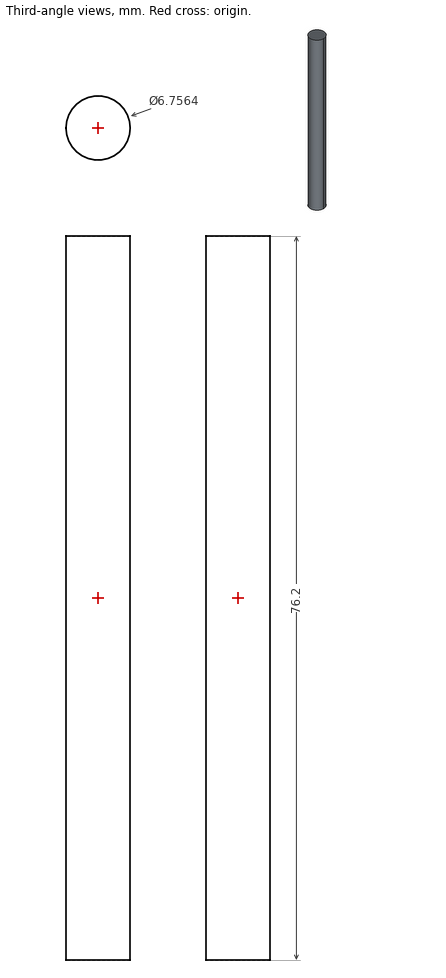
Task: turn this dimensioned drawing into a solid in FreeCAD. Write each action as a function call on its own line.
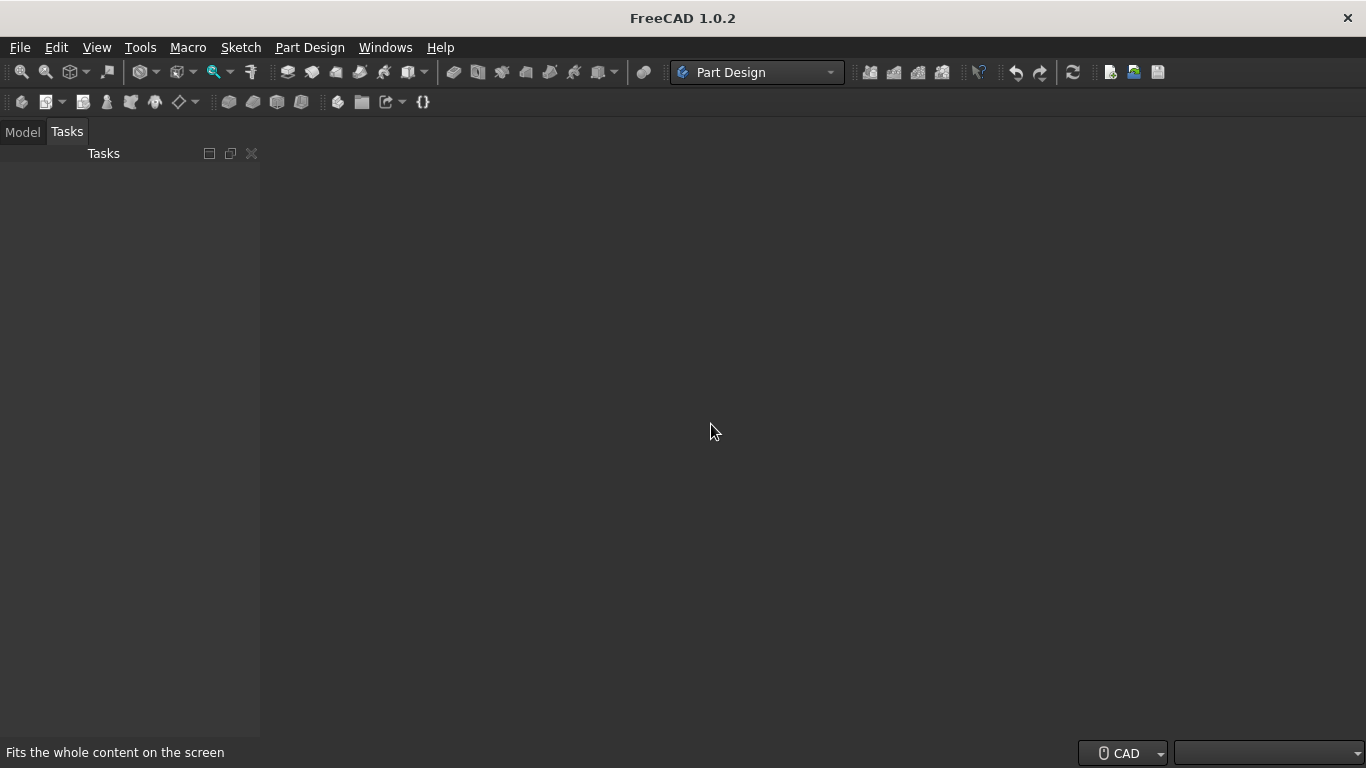
click(1110, 72)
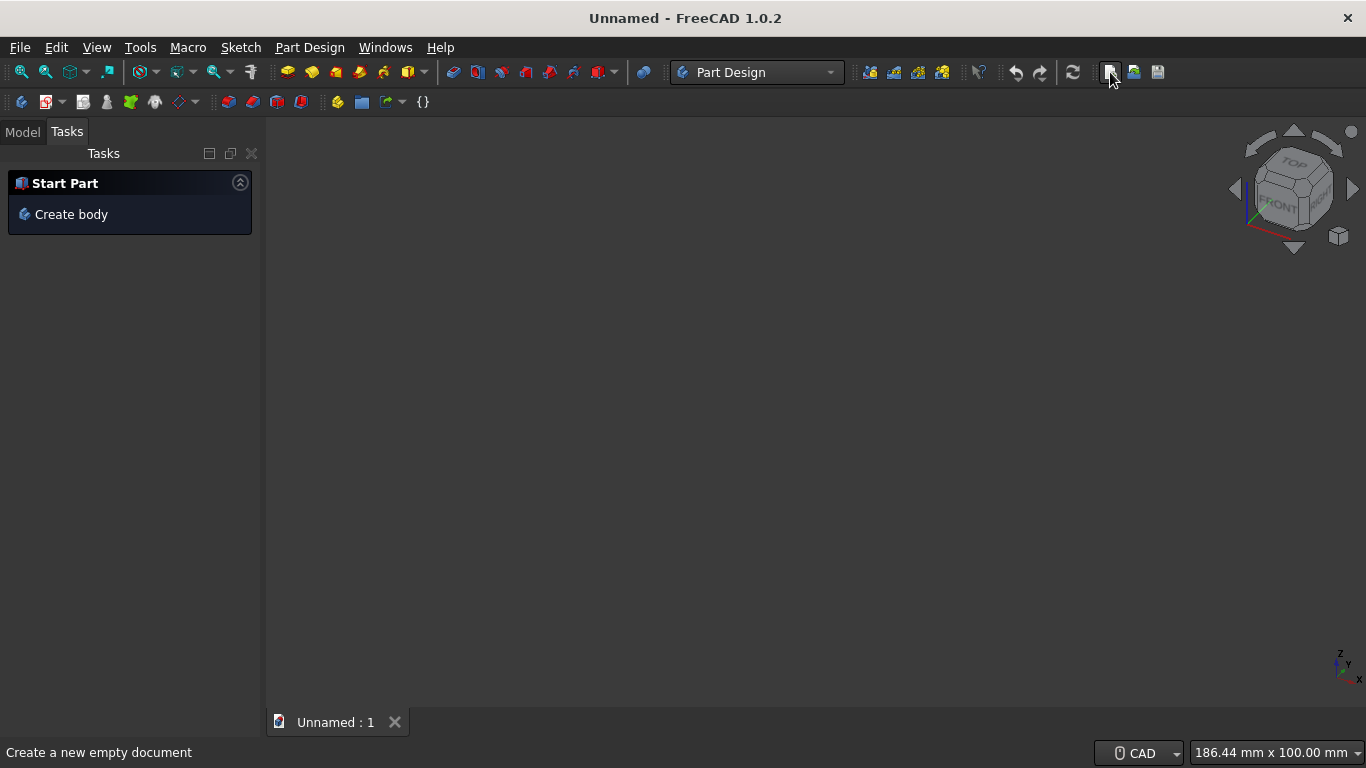
click(46, 102)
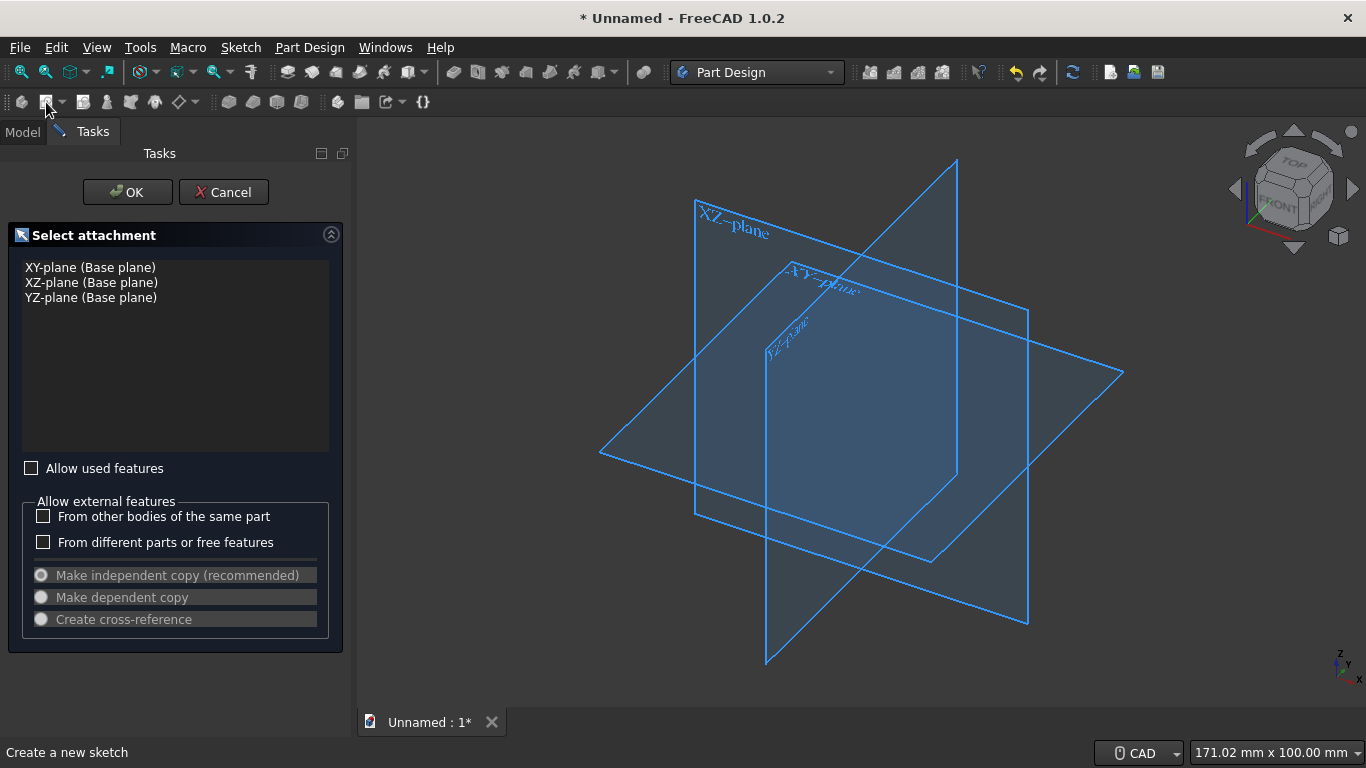
click(82, 268)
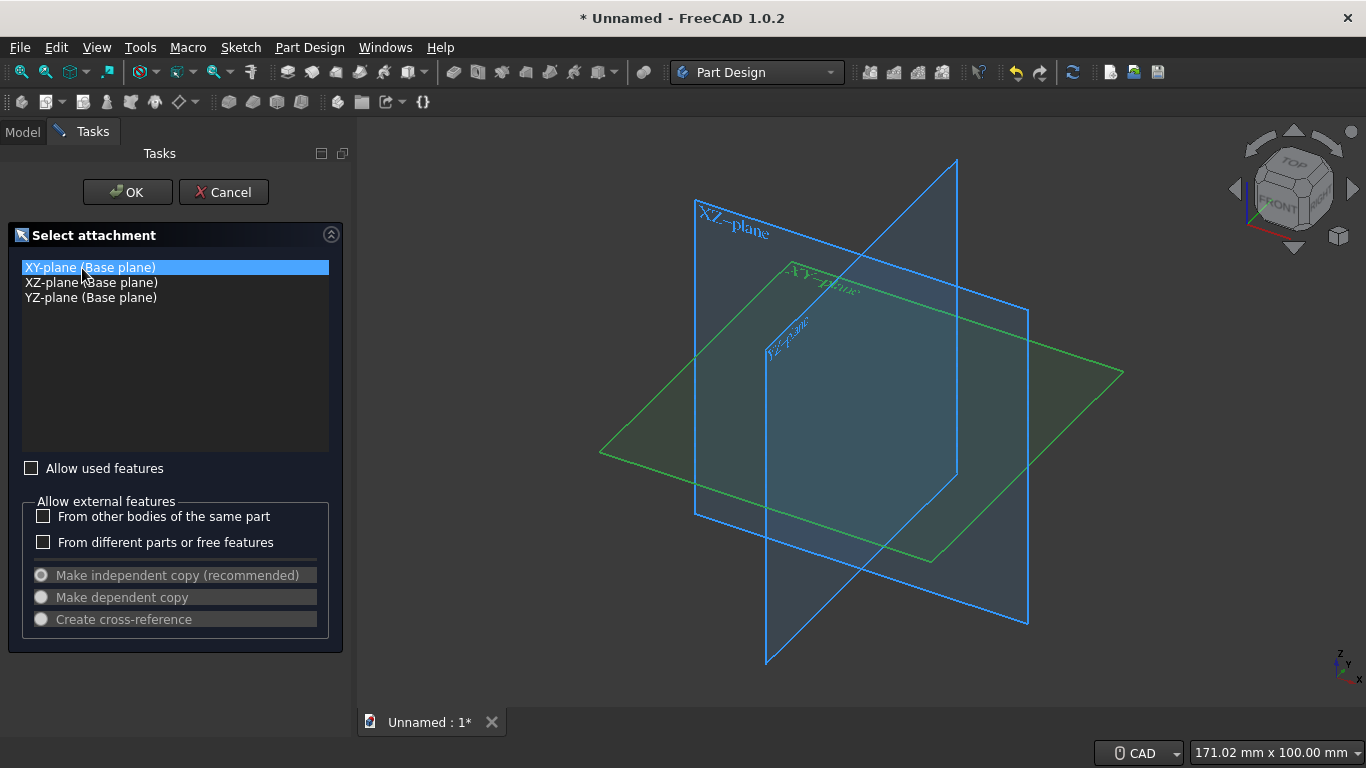
click(128, 192)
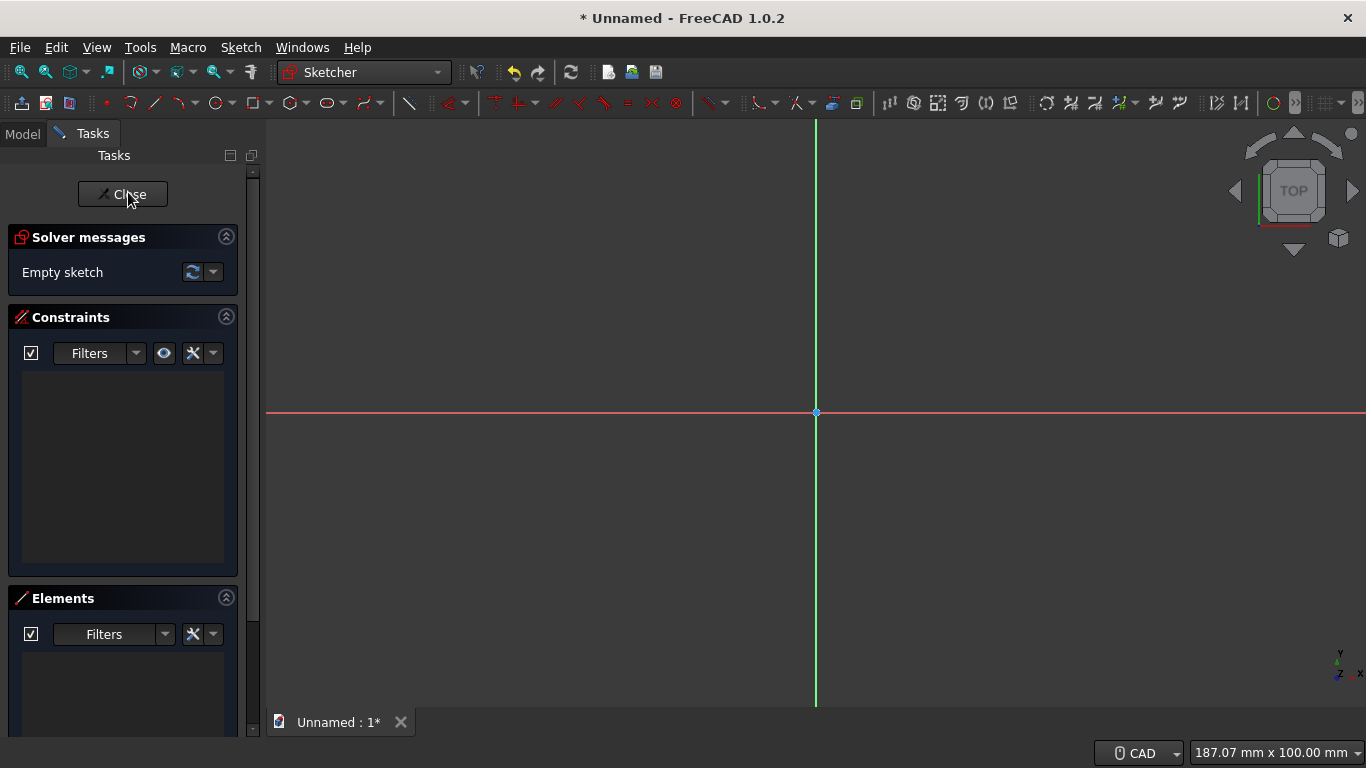
scroll(825, 413, up, 11)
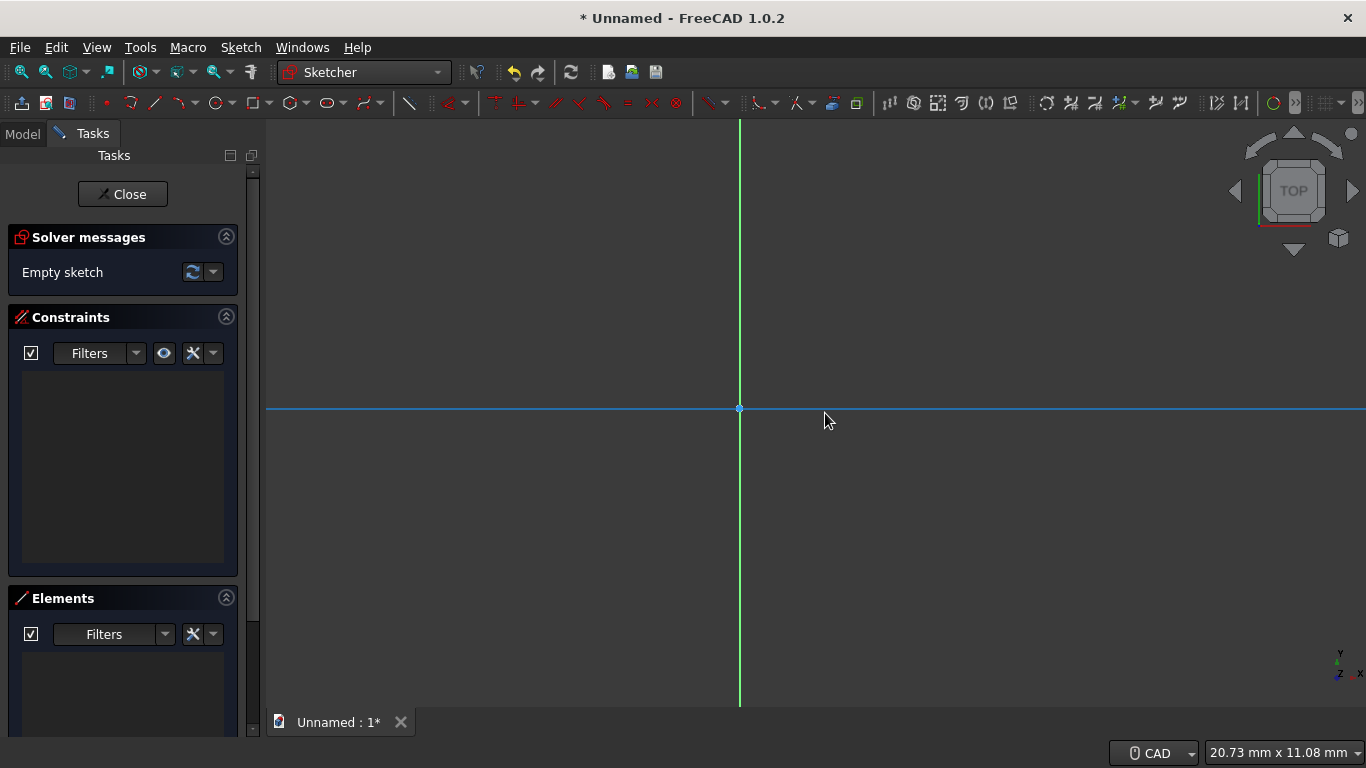
click(216, 104)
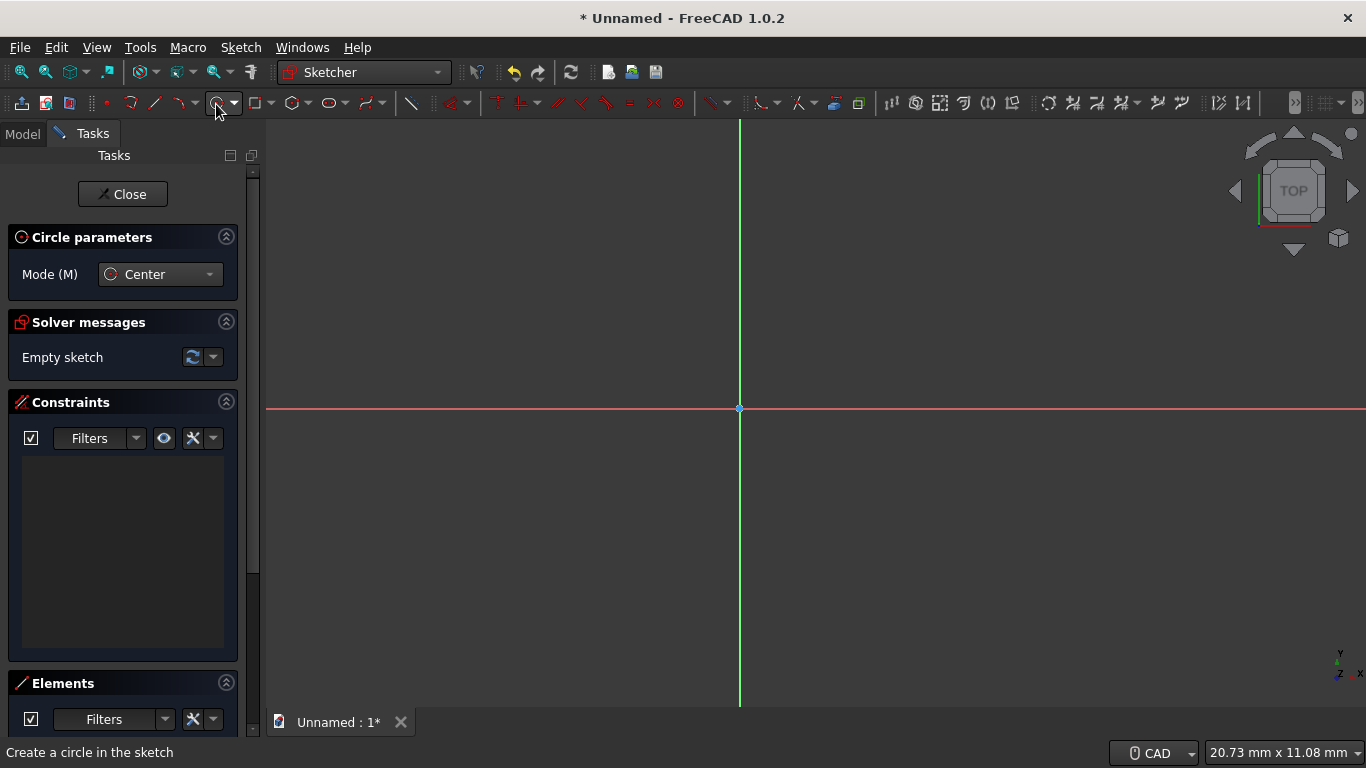
click(740, 409)
move(866, 282)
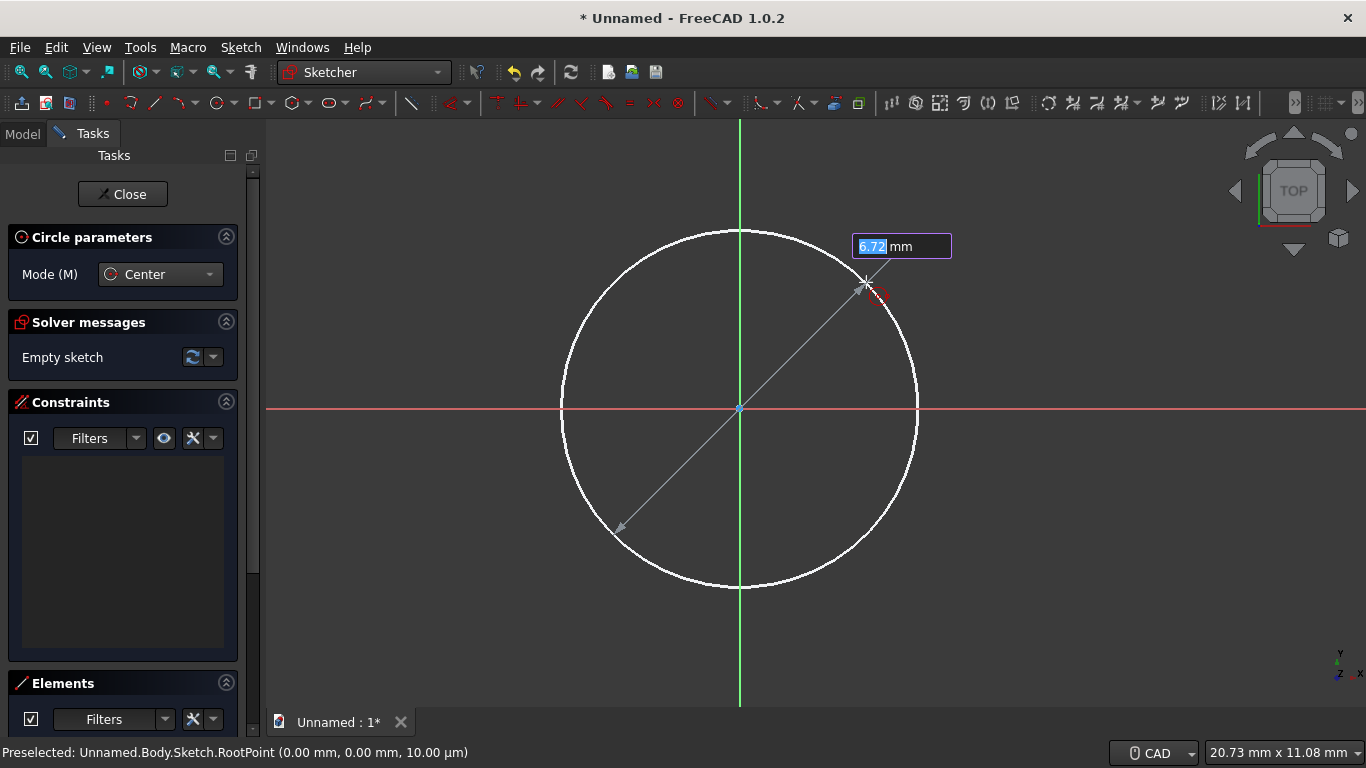
text(6.7564)
key(Return)
key(Escape)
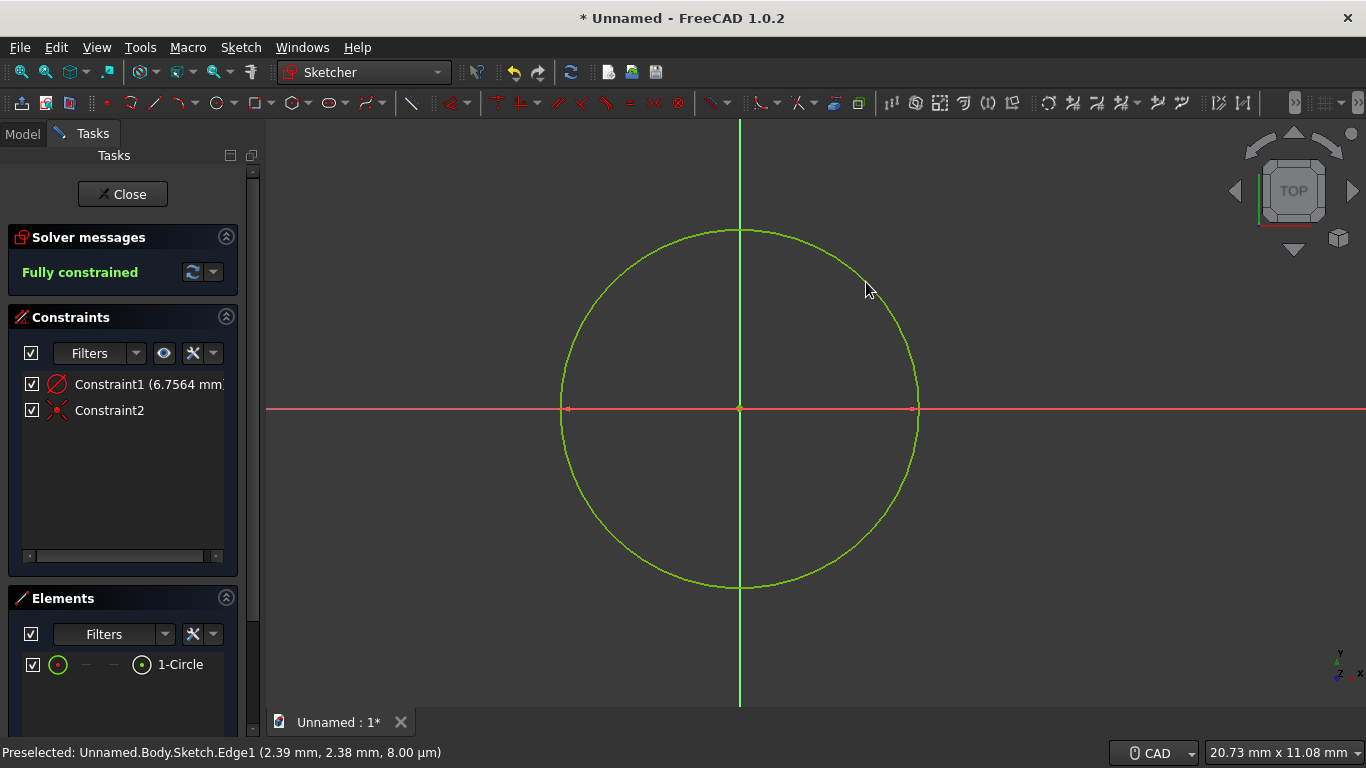
click(123, 194)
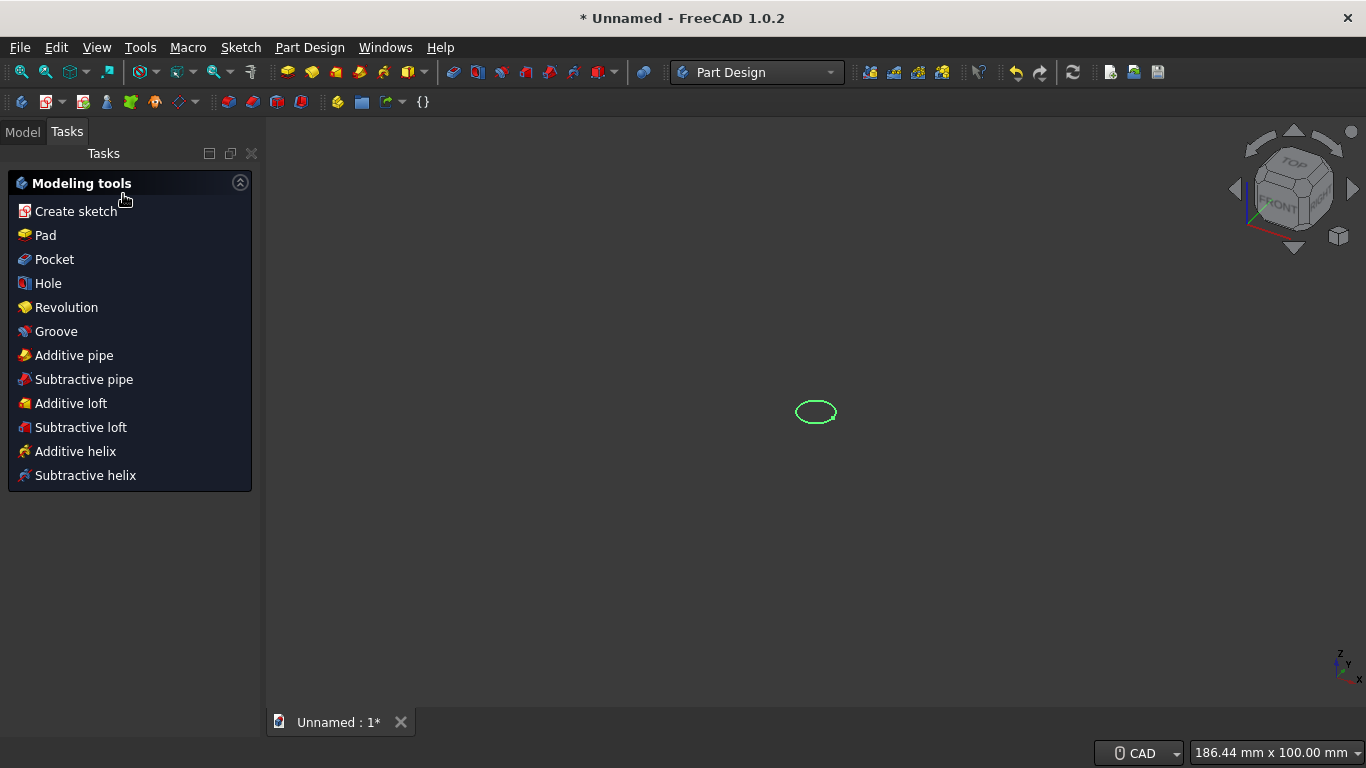
click(288, 72)